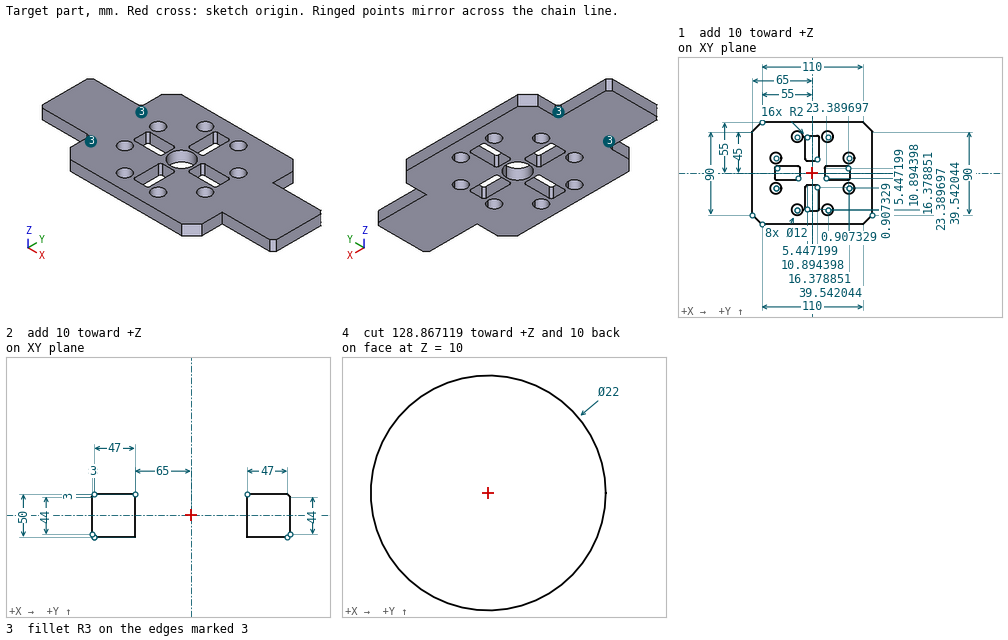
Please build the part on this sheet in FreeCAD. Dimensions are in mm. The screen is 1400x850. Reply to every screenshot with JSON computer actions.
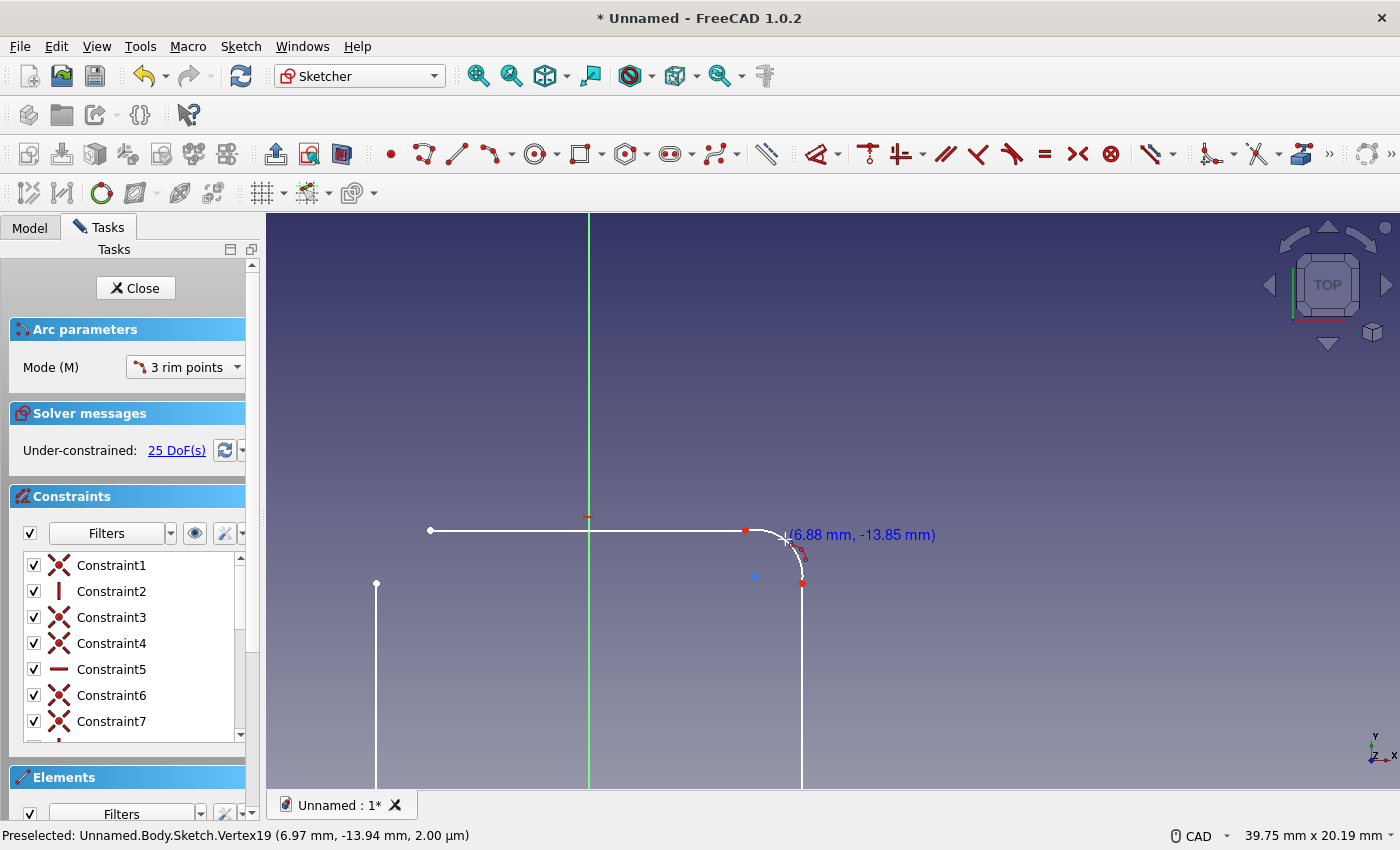
{"action": "scroll", "coordinate": [786, 545], "scroll_direction": "down", "scroll_amount": 11}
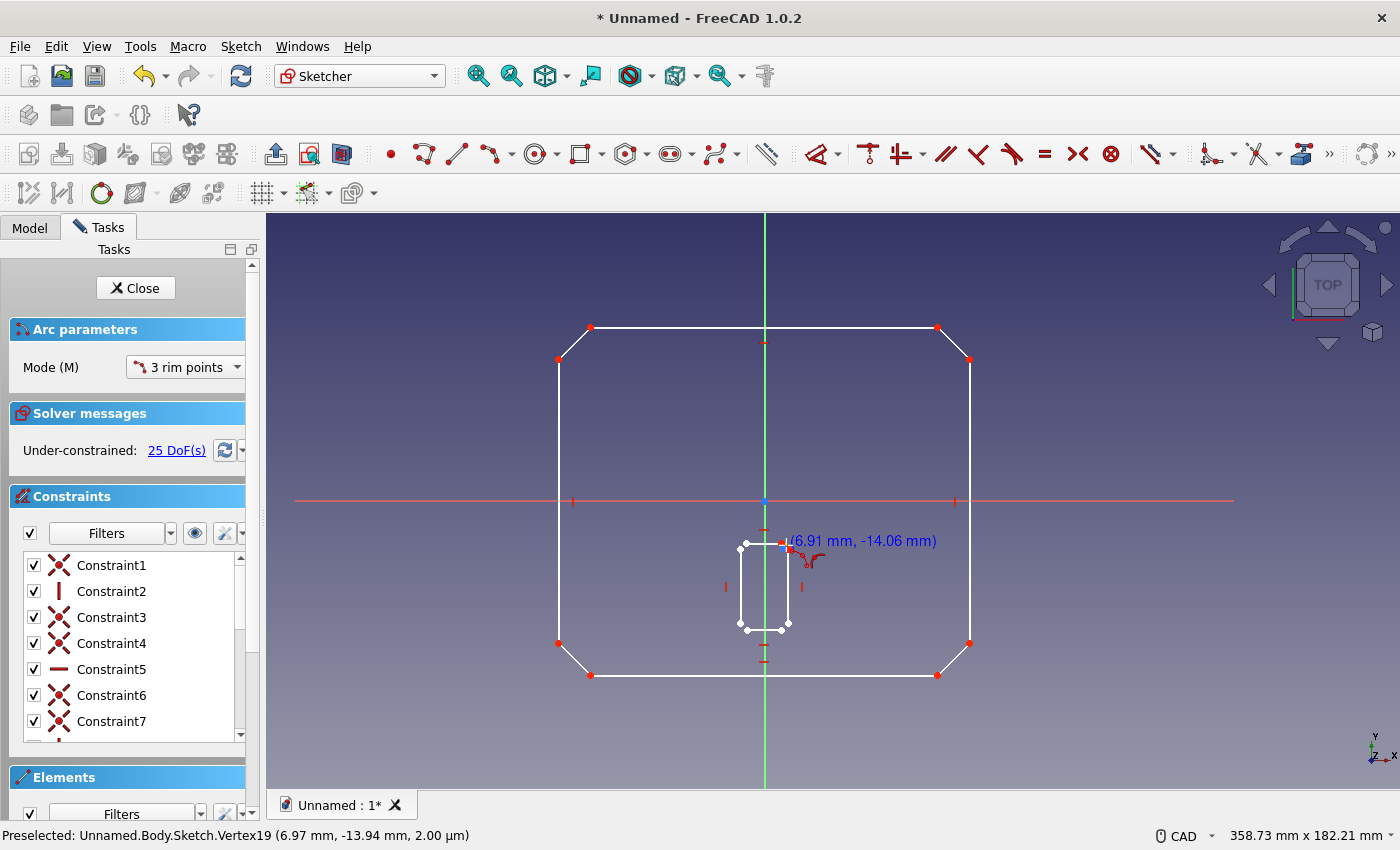
{"action": "scroll", "coordinate": [788, 623], "scroll_direction": "up", "scroll_amount": 3}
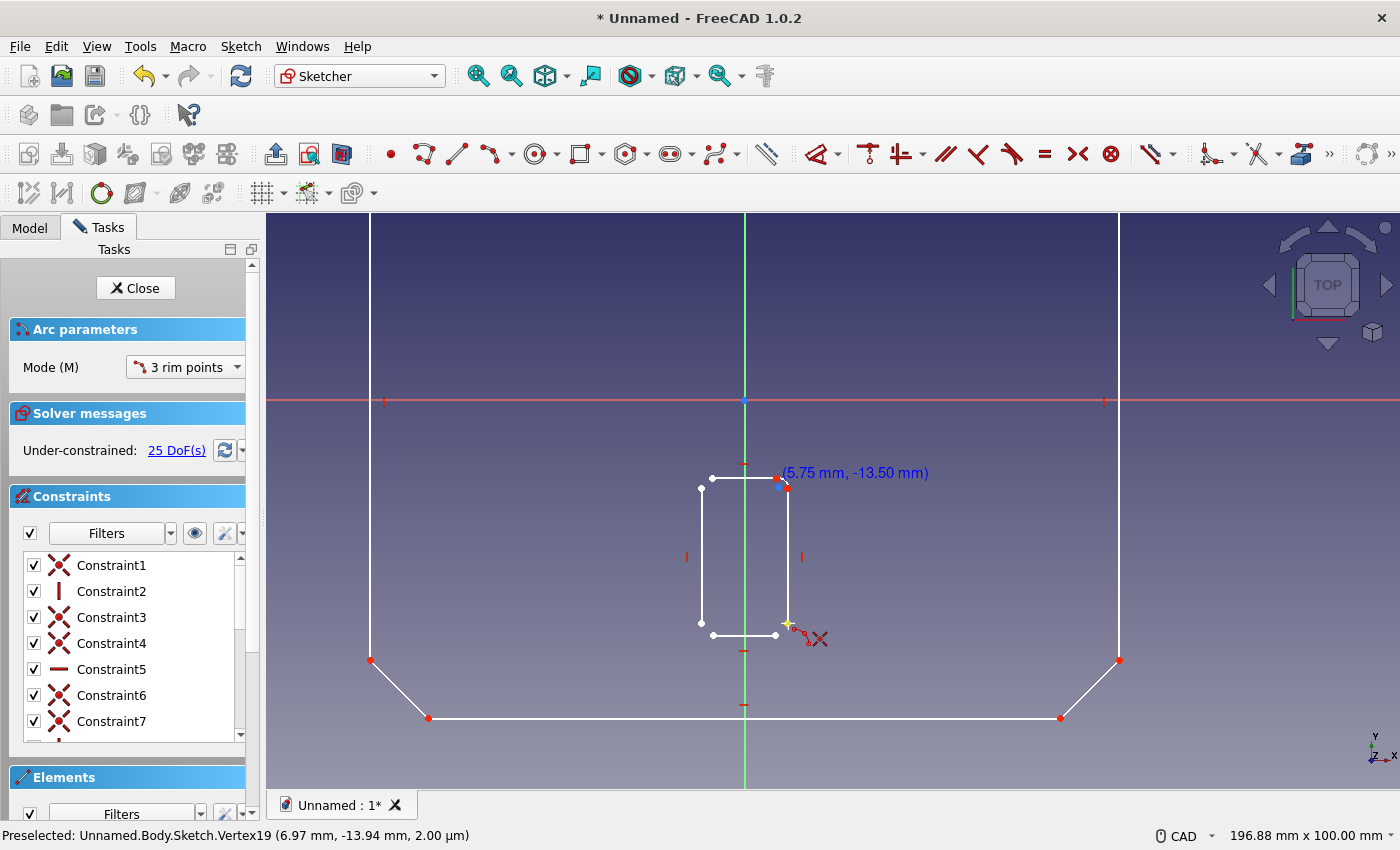
{"action": "left_click", "coordinate": [788, 624]}
{"action": "left_click", "coordinate": [776, 636]}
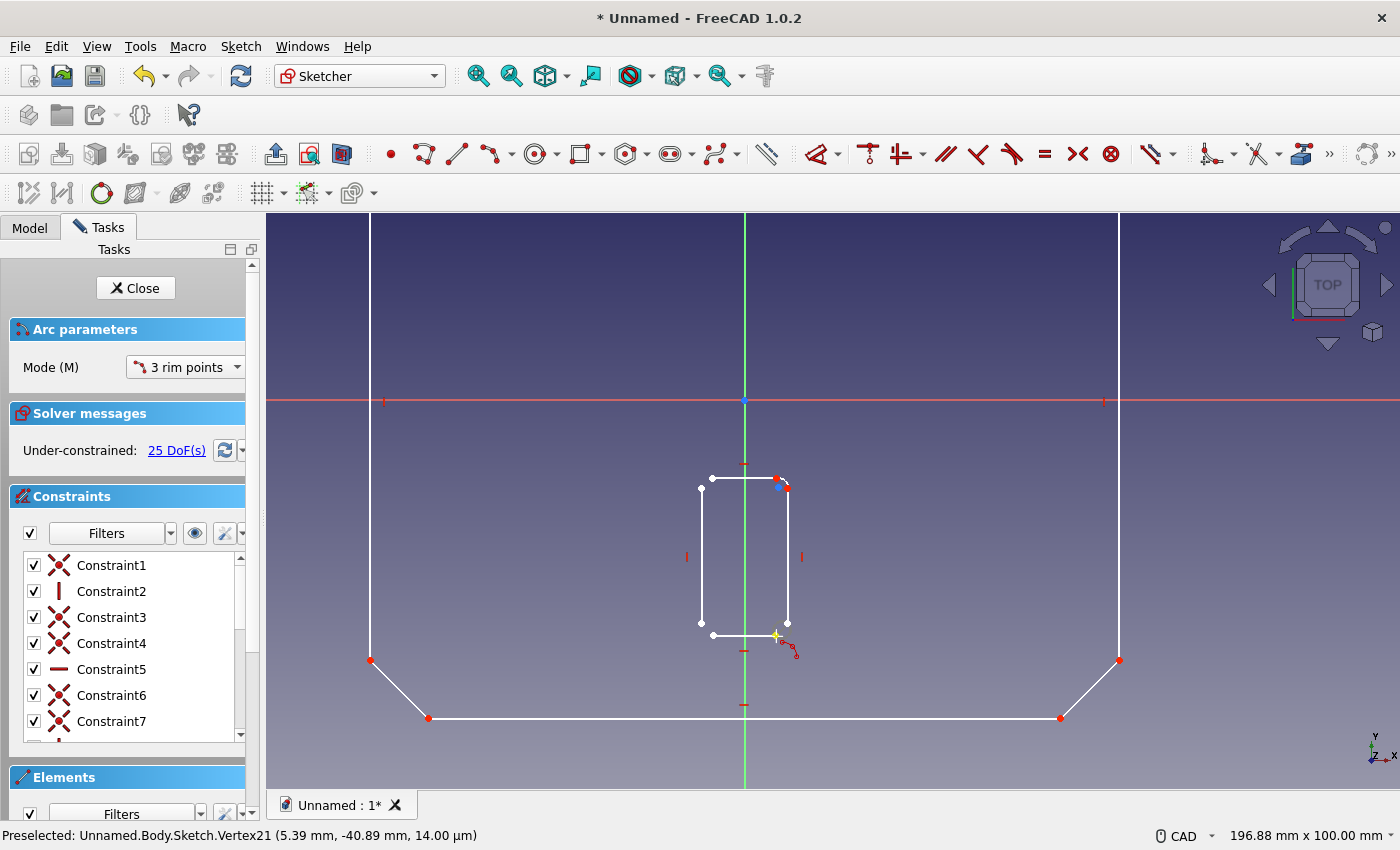
{"action": "scroll", "coordinate": [784, 631], "scroll_direction": "up", "scroll_amount": 8}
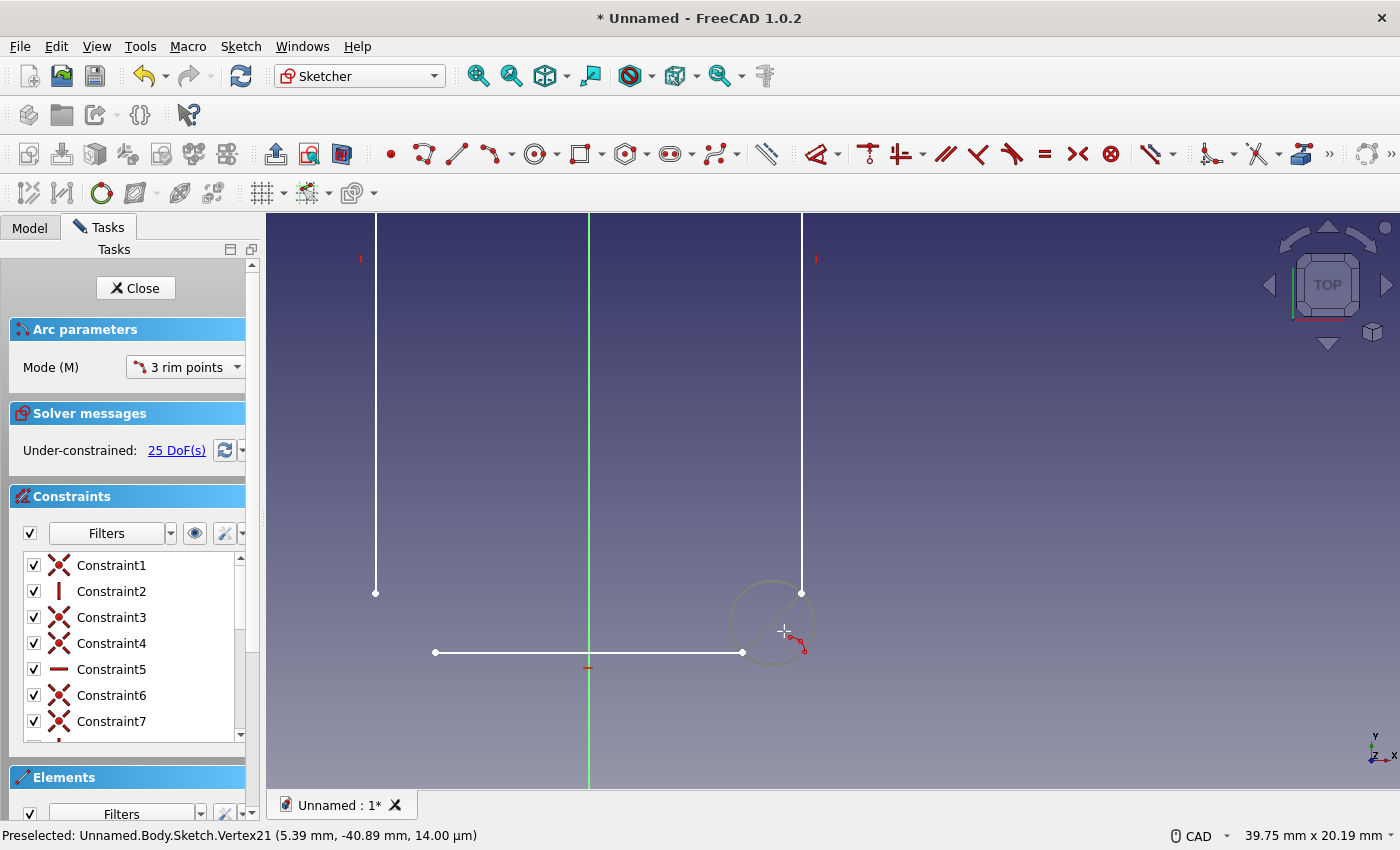
{"action": "left_click", "coordinate": [784, 629]}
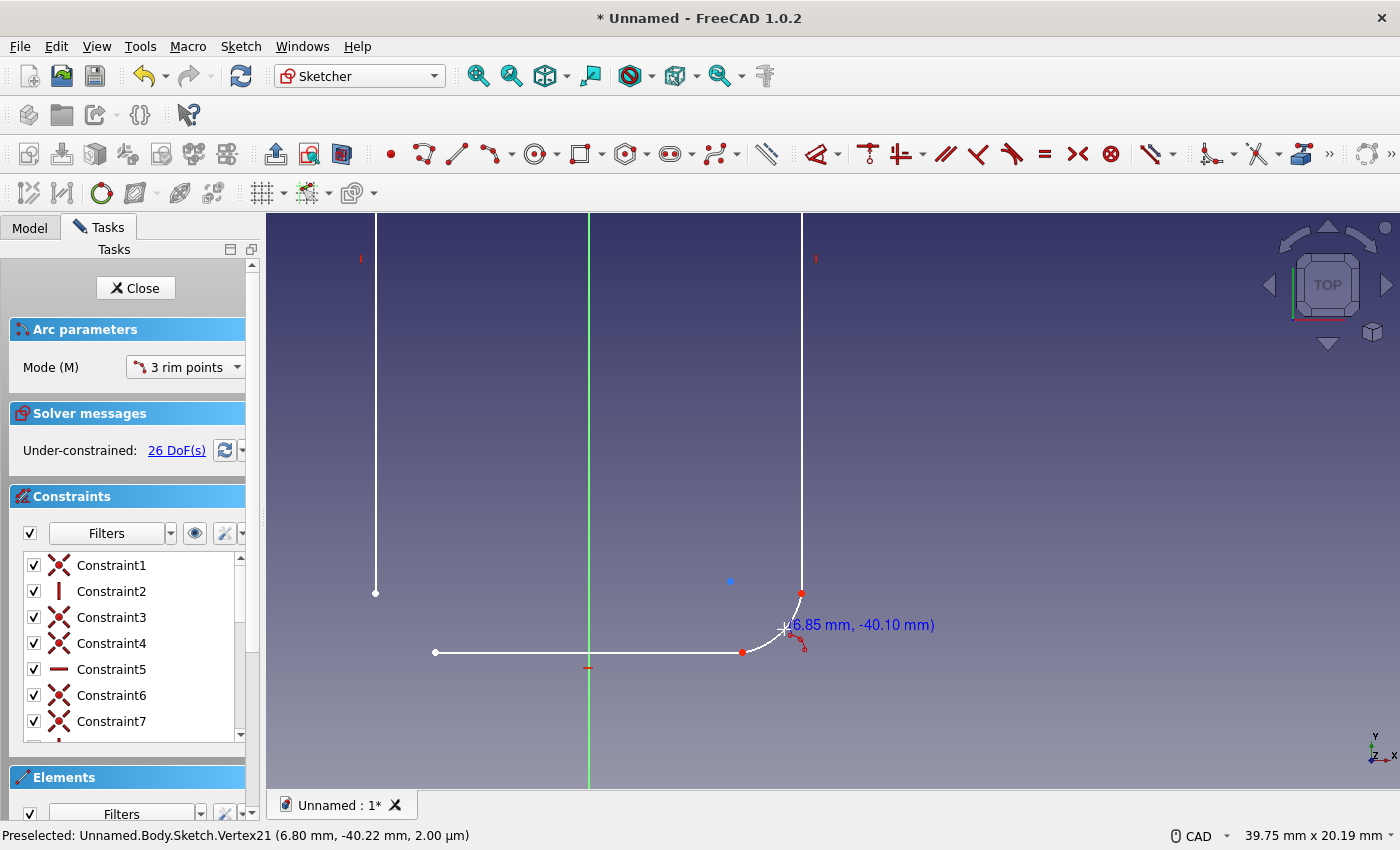
{"action": "scroll", "coordinate": [786, 627], "scroll_direction": "down", "scroll_amount": 11}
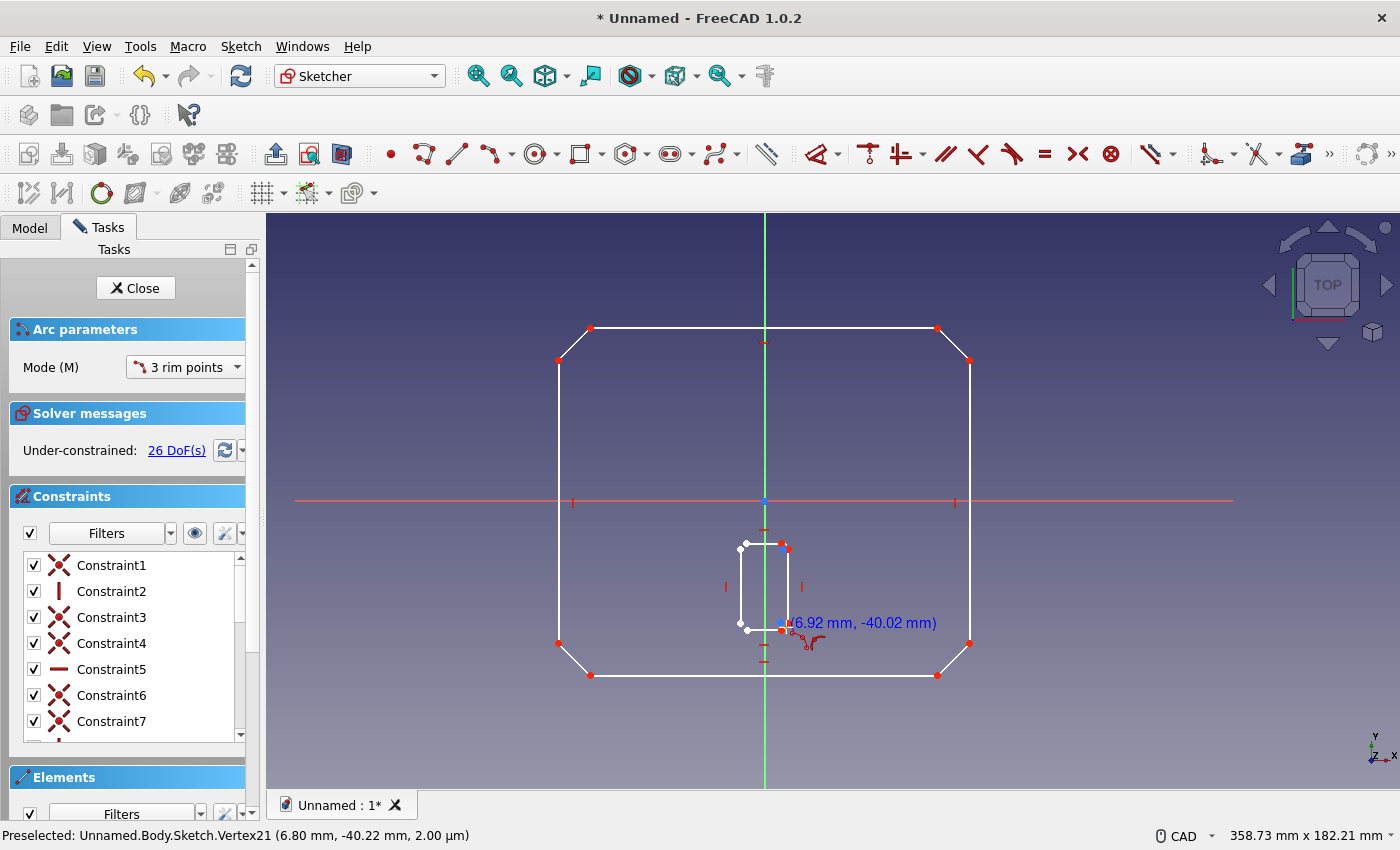
{"action": "scroll", "coordinate": [747, 630], "scroll_direction": "up", "scroll_amount": 3}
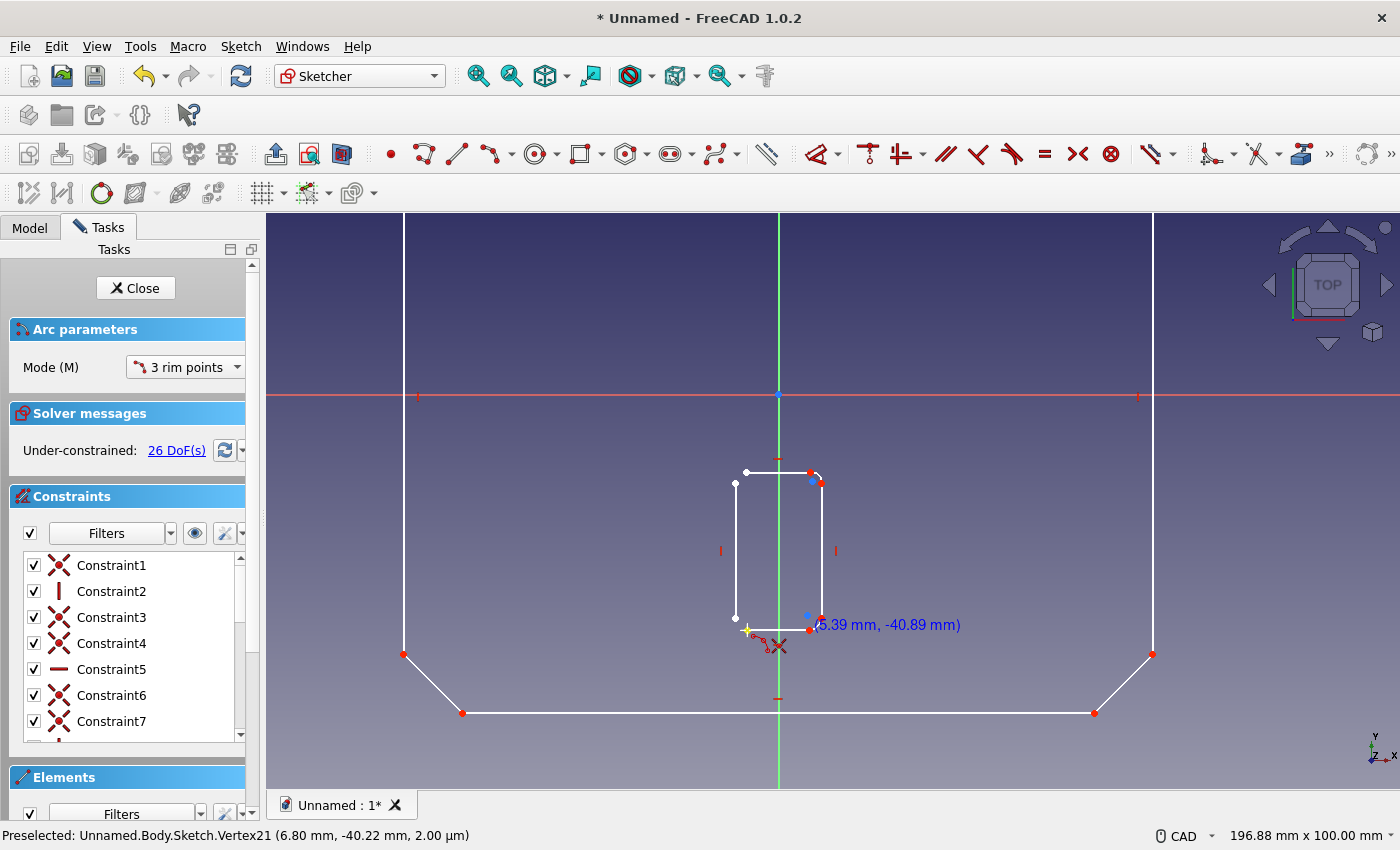
{"action": "left_click", "coordinate": [748, 630]}
{"action": "left_click", "coordinate": [736, 618]}